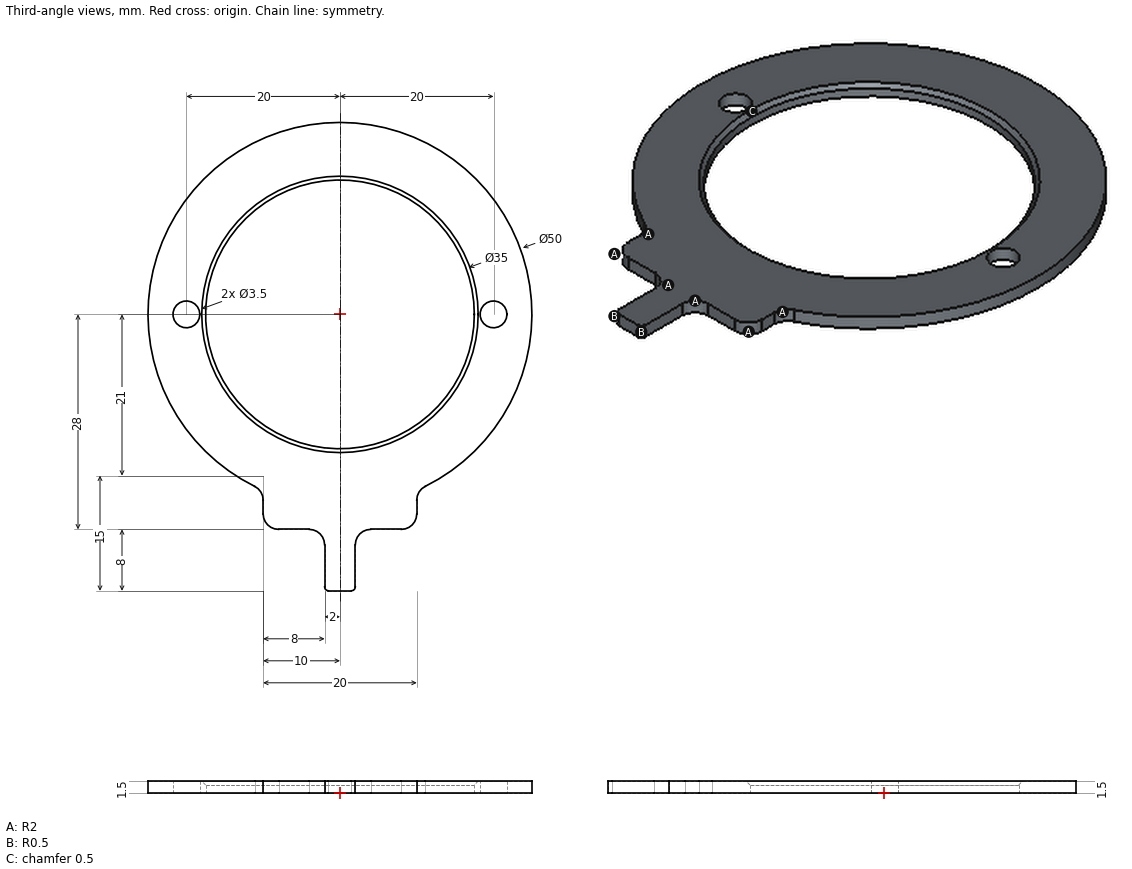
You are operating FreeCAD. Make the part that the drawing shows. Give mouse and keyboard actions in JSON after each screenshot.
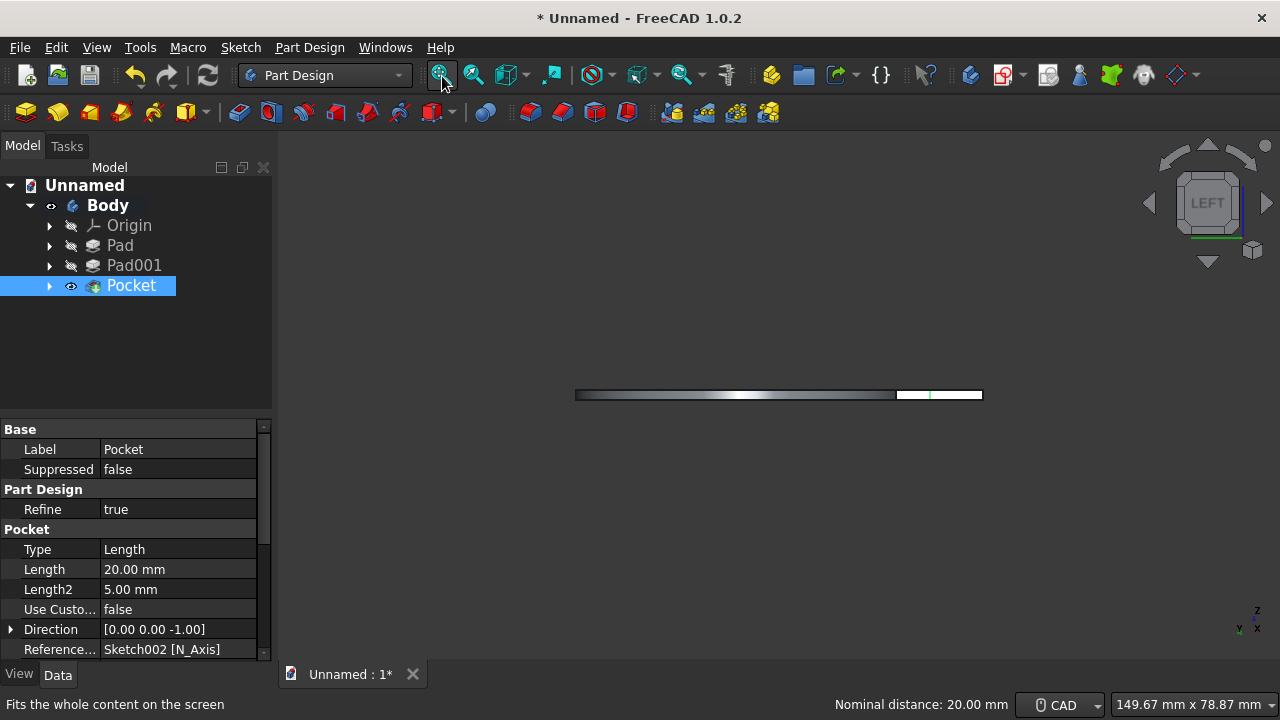
{"action": "key", "text": "v 3"}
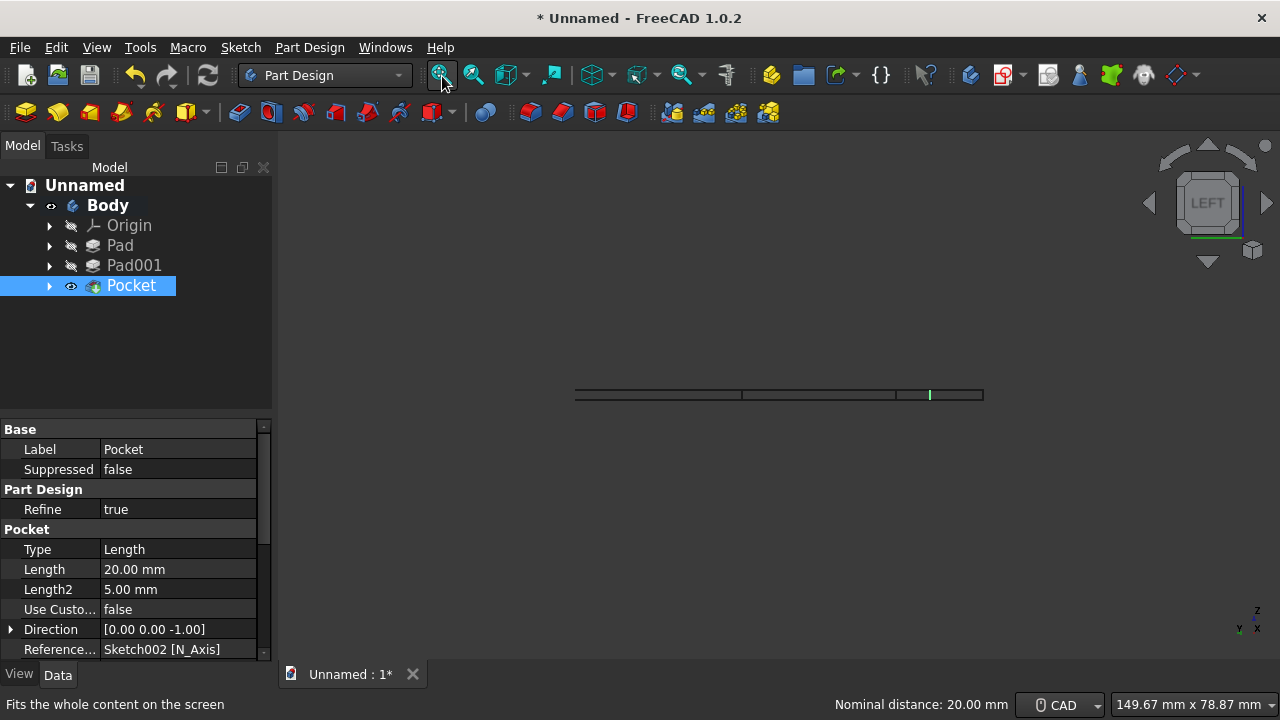
{"action": "key", "text": "0"}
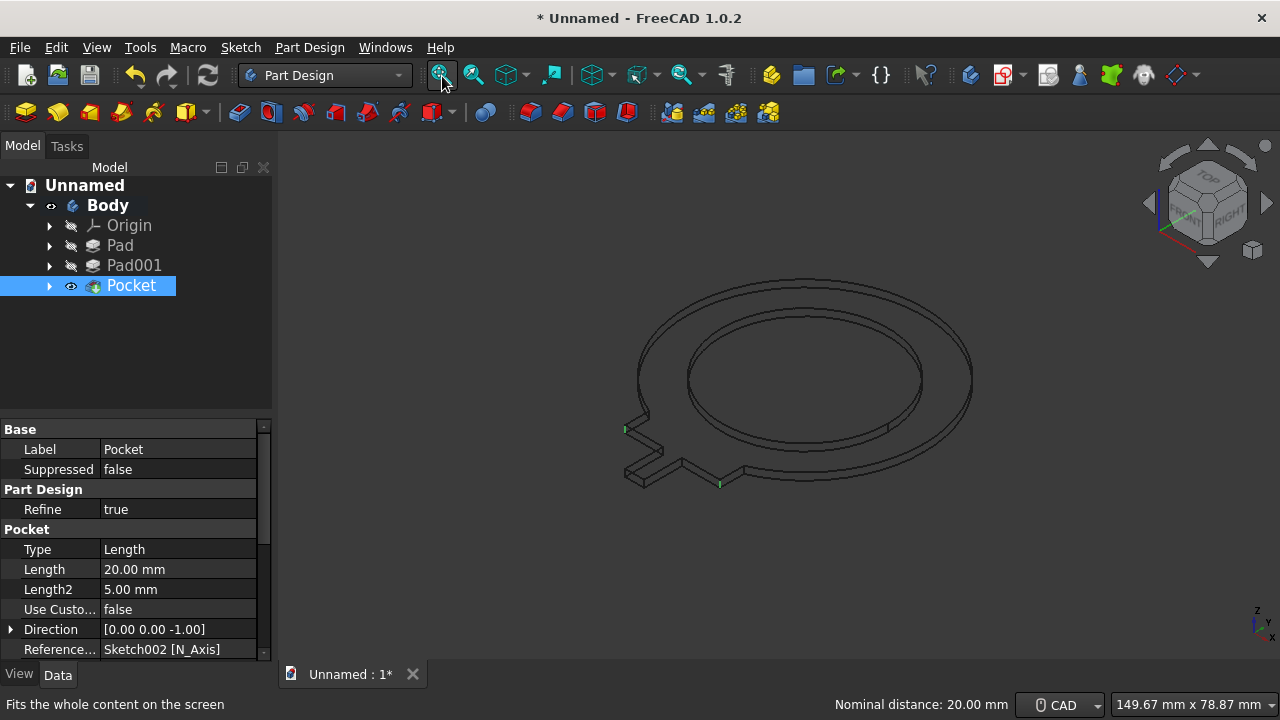
{"action": "scroll", "coordinate": [744, 469], "scroll_direction": "up", "scroll_amount": 7}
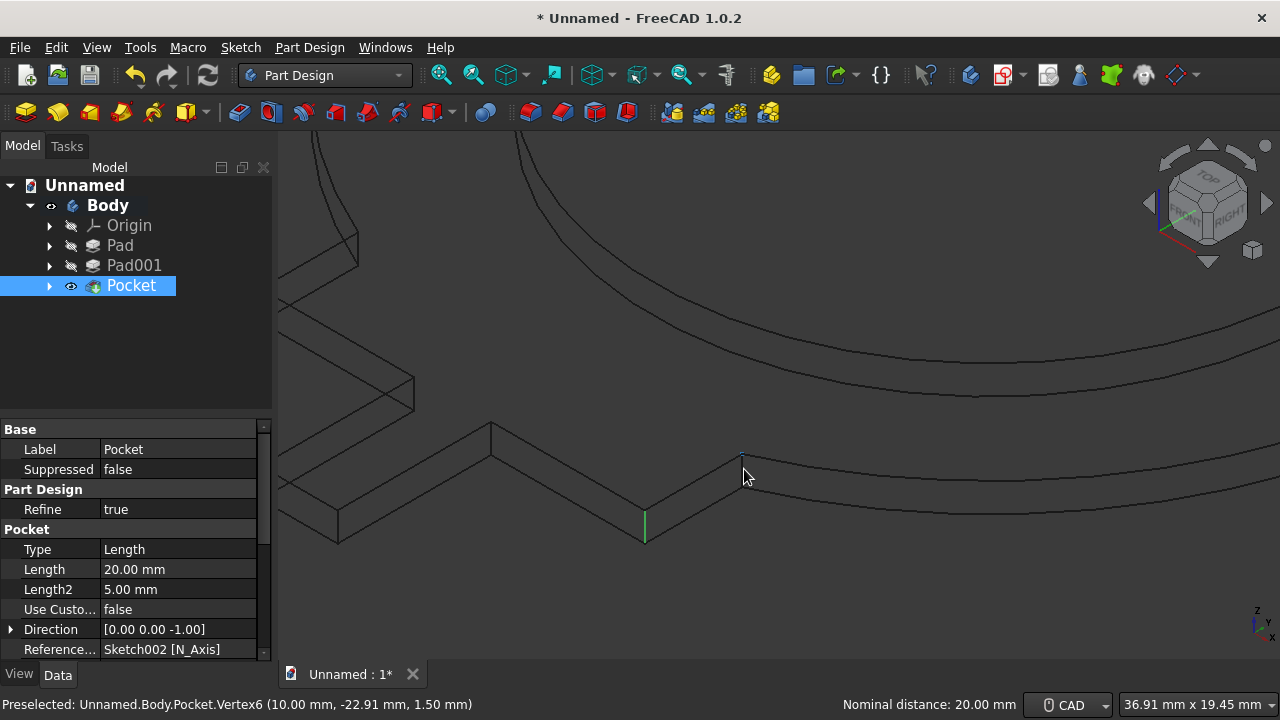
{"action": "left_click", "coordinate": [742, 470], "text": "ctrl"}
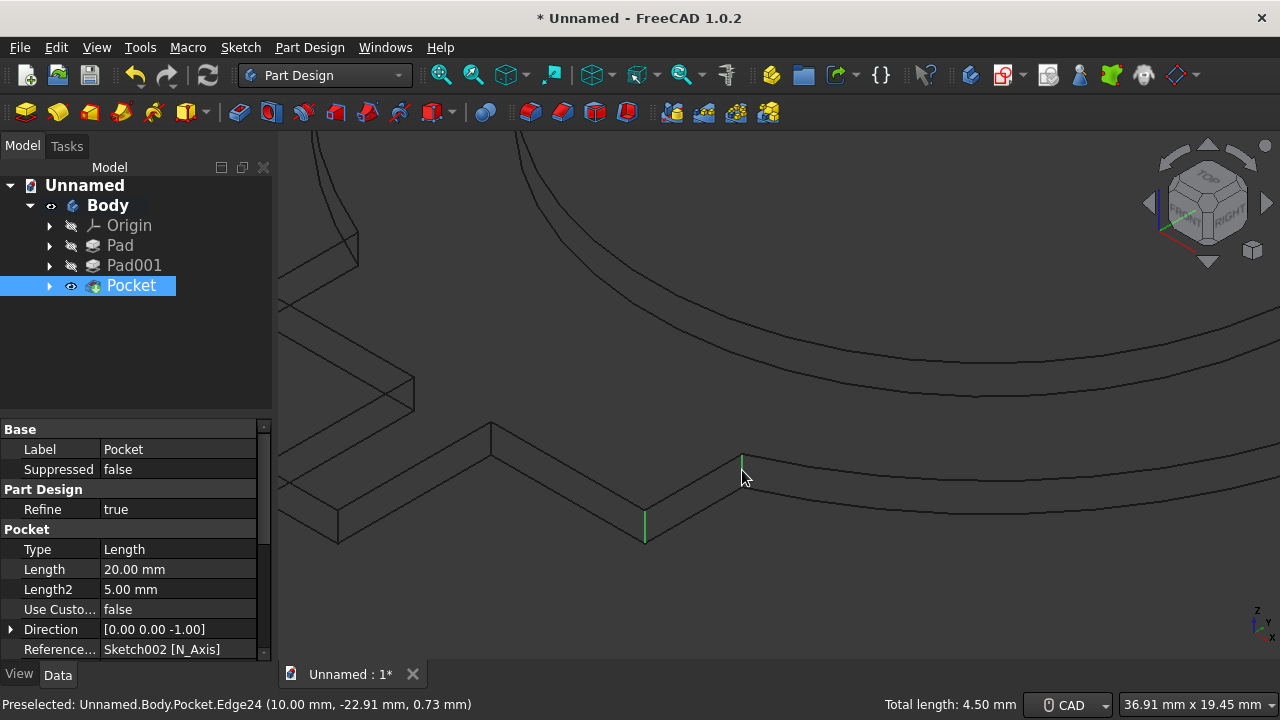
{"action": "left_click", "coordinate": [358, 248], "text": "ctrl"}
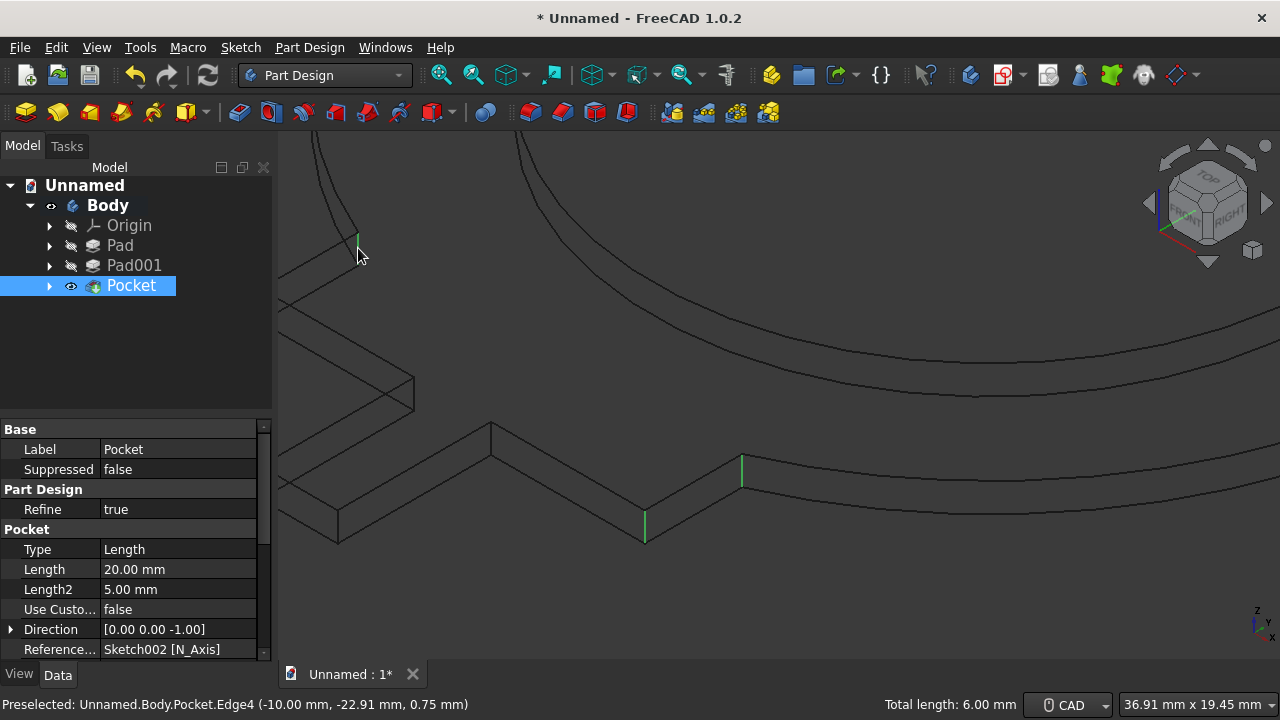
{"action": "left_click", "coordinate": [414, 393], "text": "ctrl"}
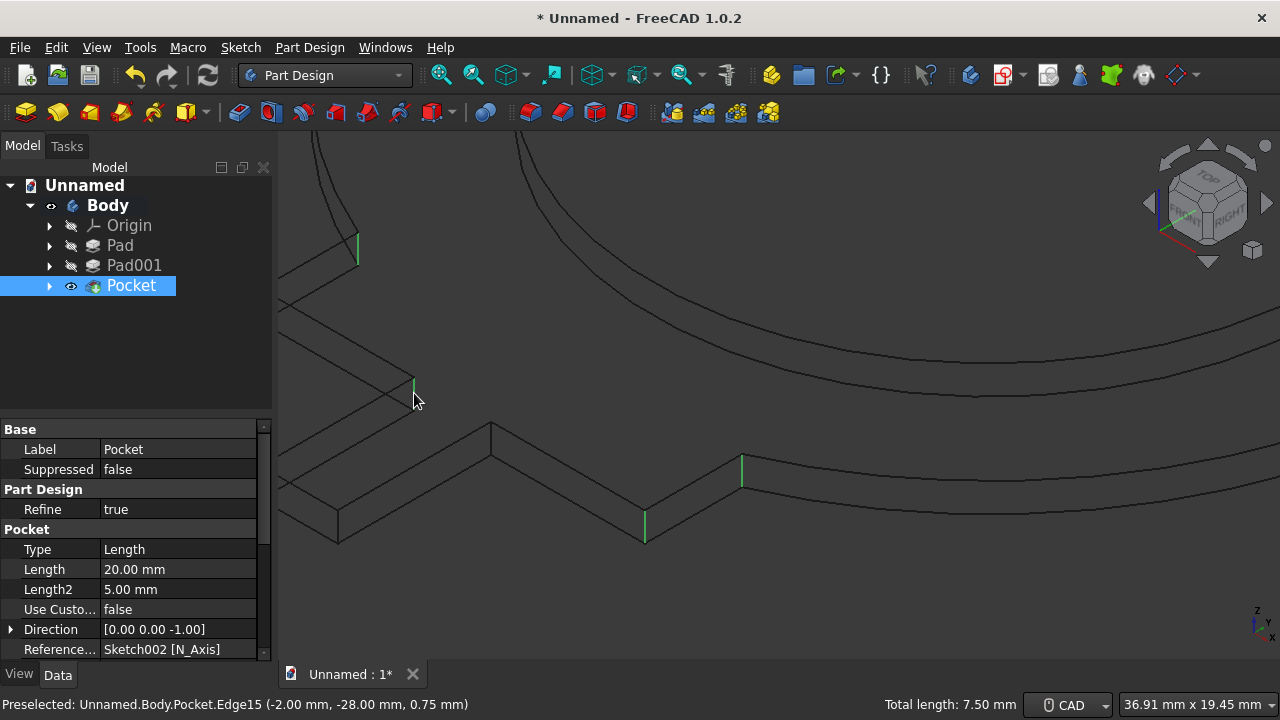
{"action": "left_click", "coordinate": [491, 437], "text": "ctrl"}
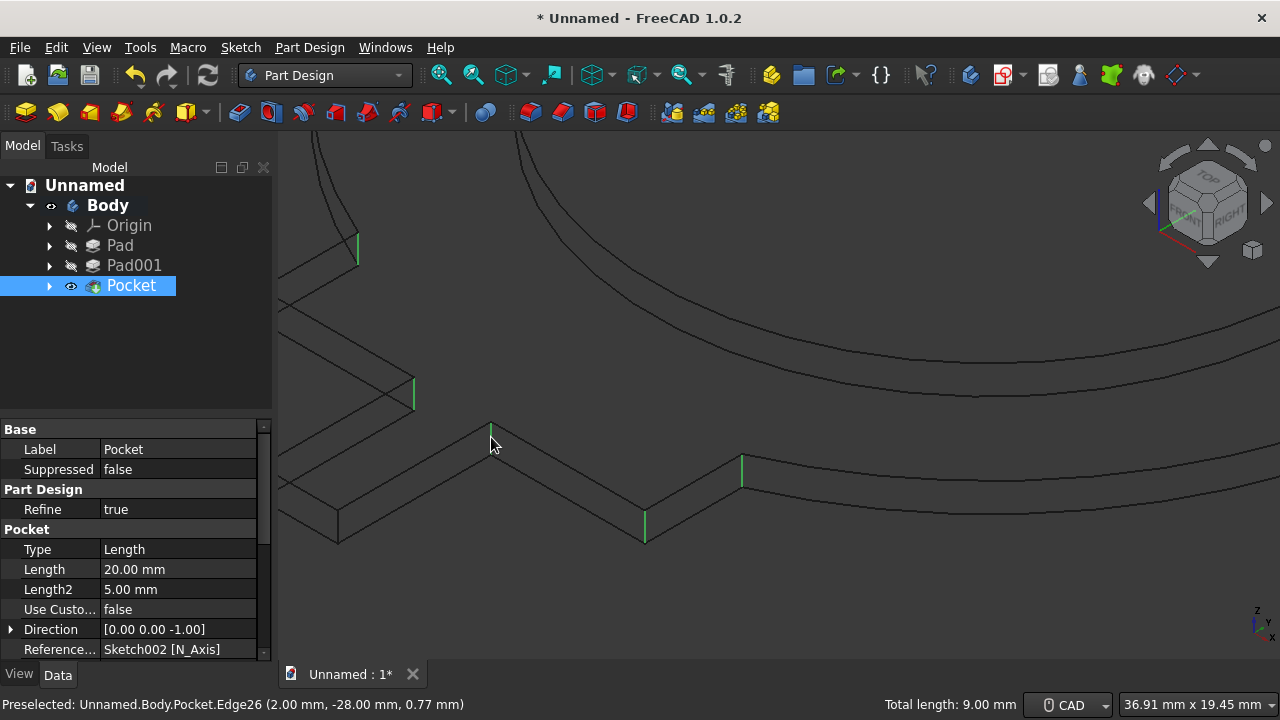
{"action": "key", "text": "v 1"}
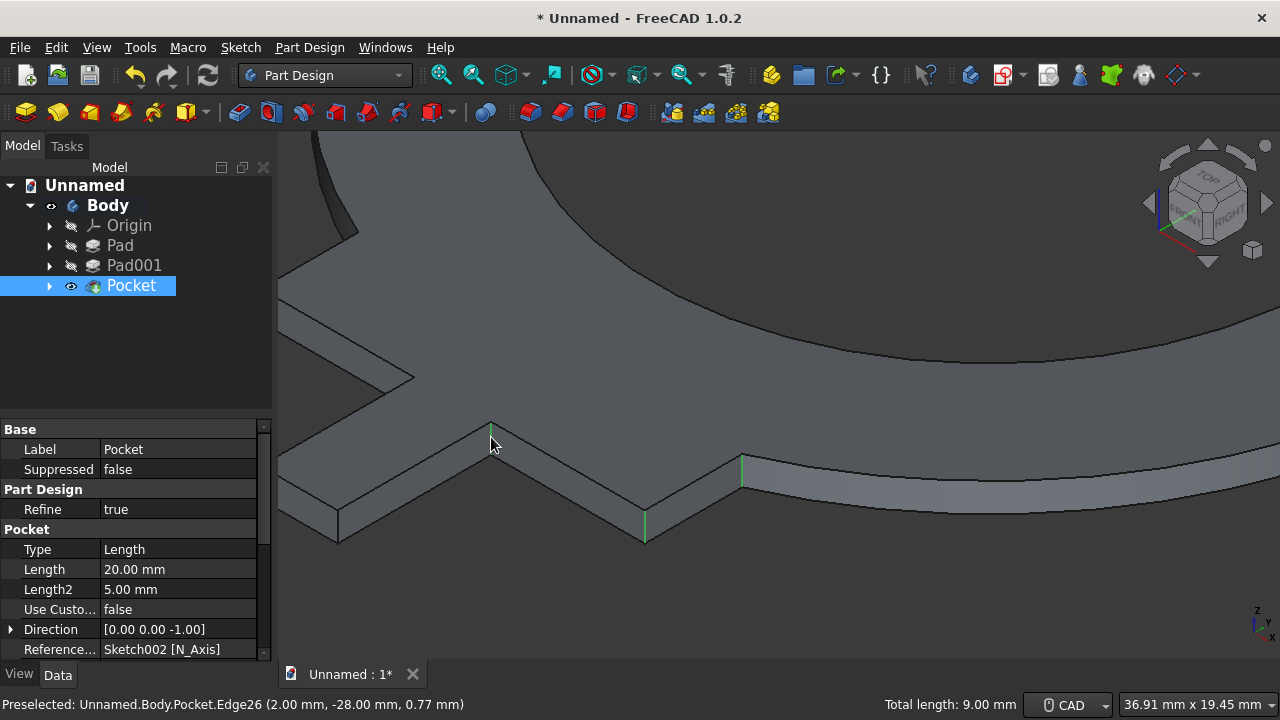
{"action": "left_click", "coordinate": [532, 112]}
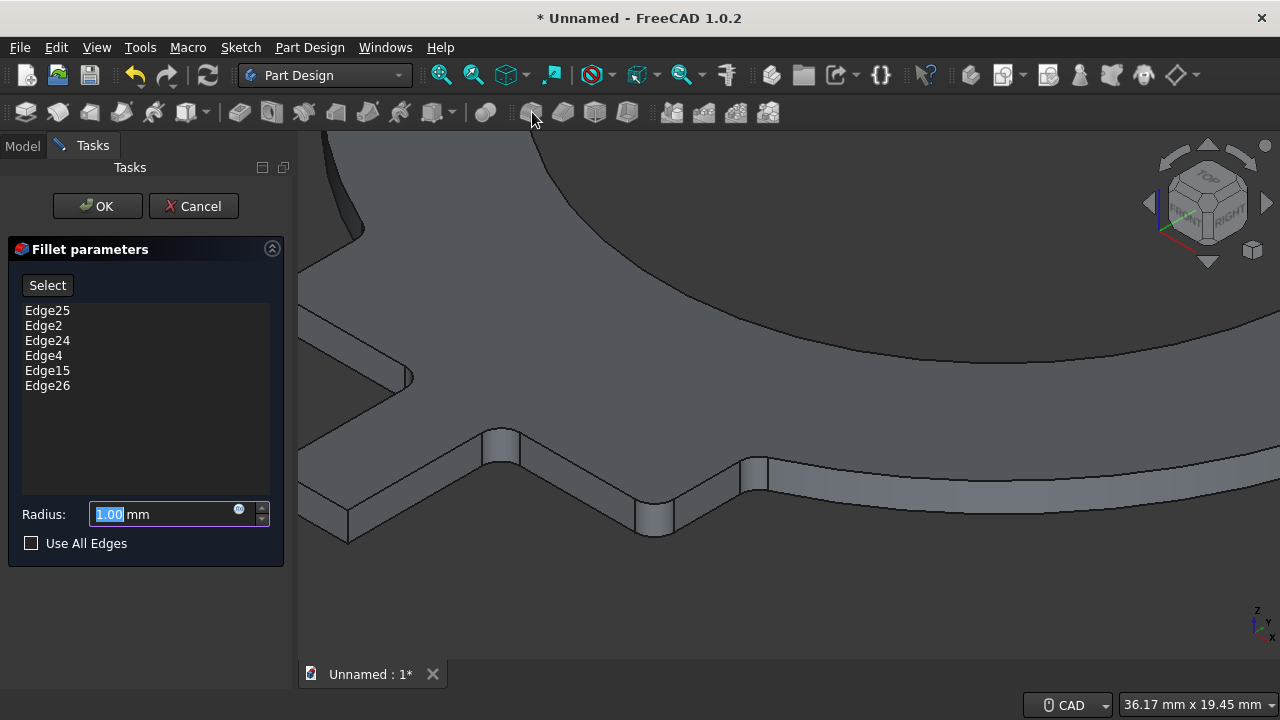
{"action": "type", "text": "2"}
{"action": "key", "text": "Tab"}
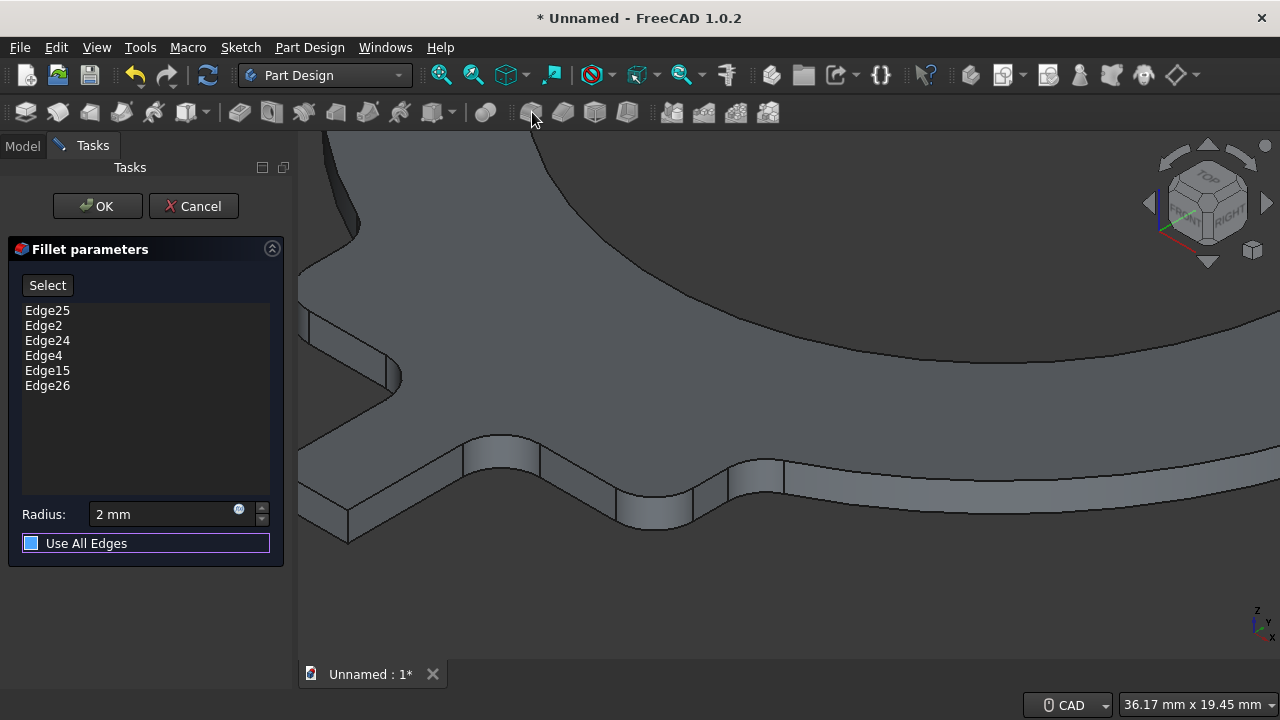
{"action": "left_click", "coordinate": [98, 206]}